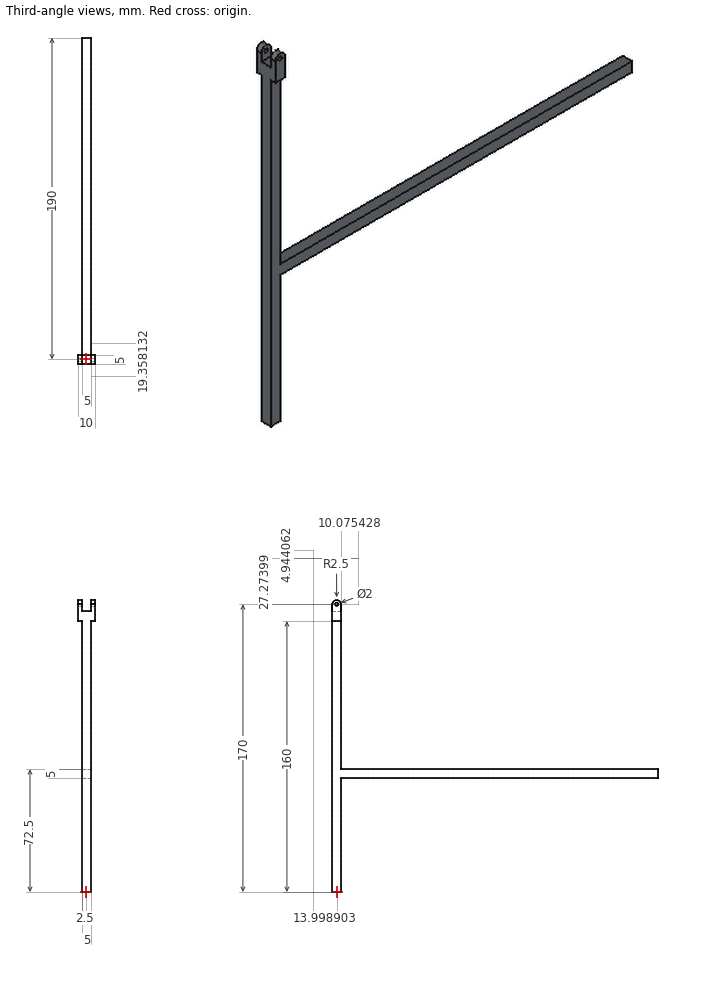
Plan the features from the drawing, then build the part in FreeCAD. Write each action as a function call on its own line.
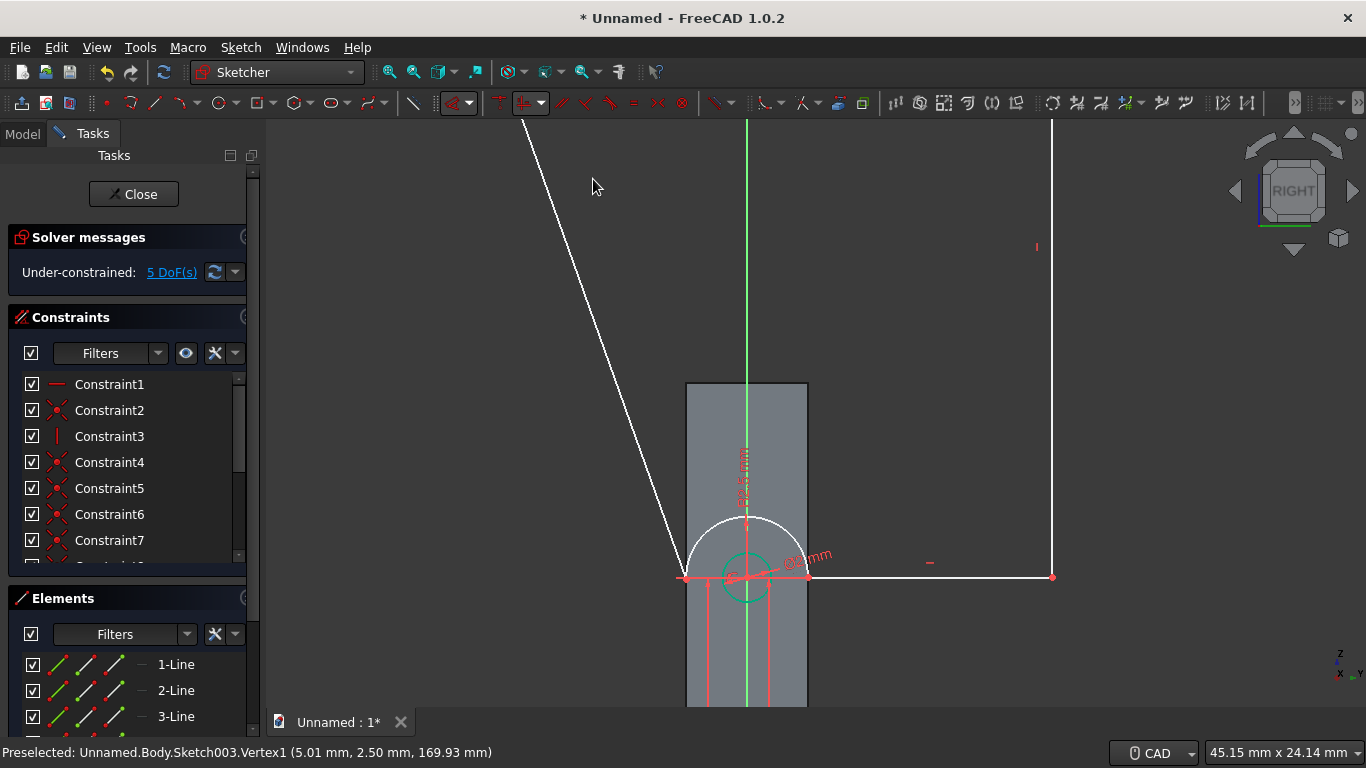
click(686, 579)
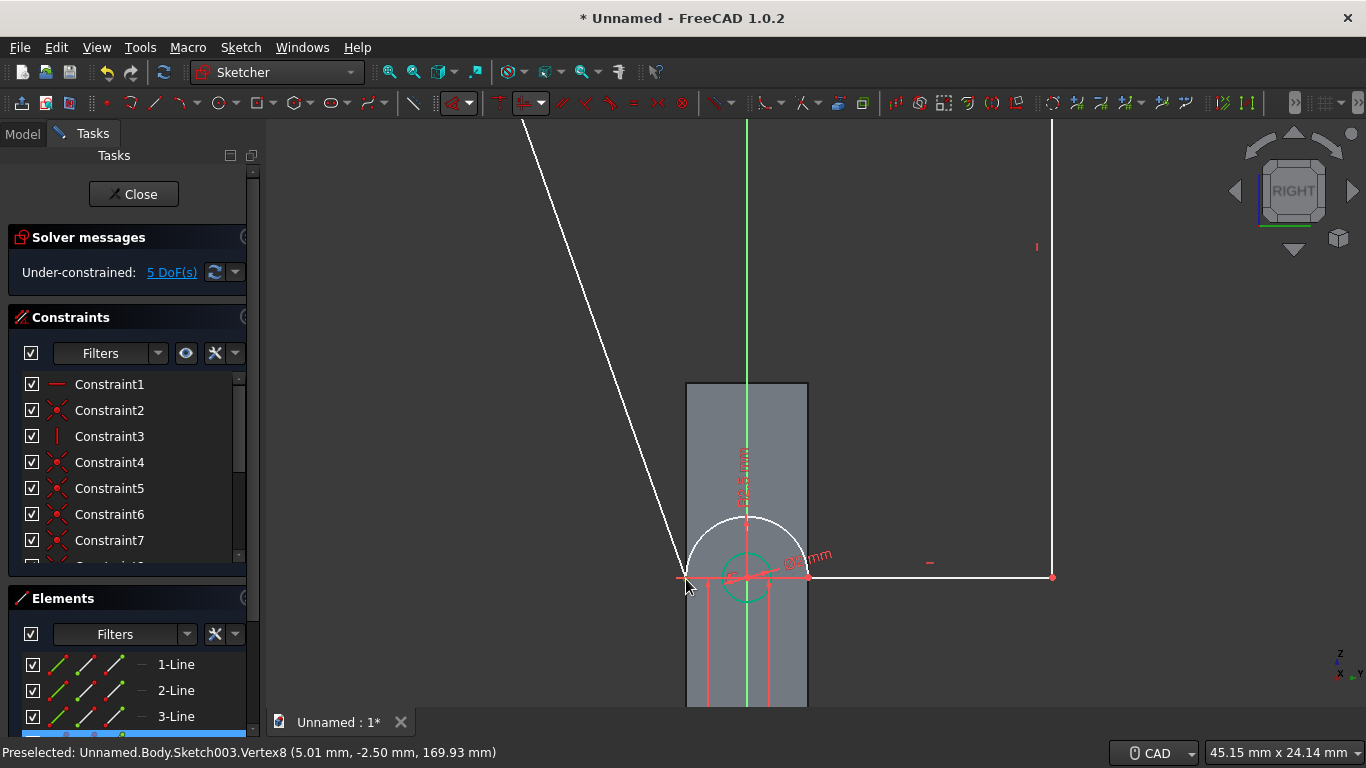
click(472, 104)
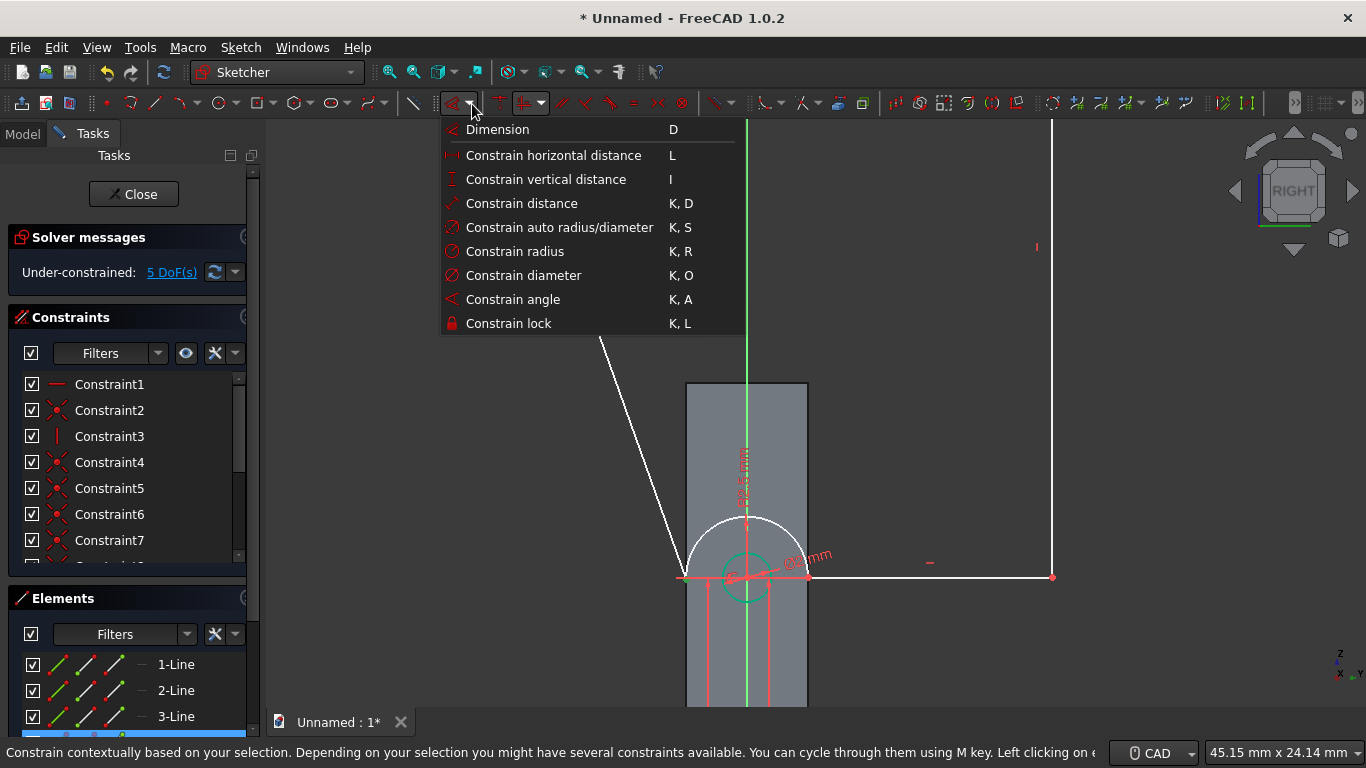
click(593, 179)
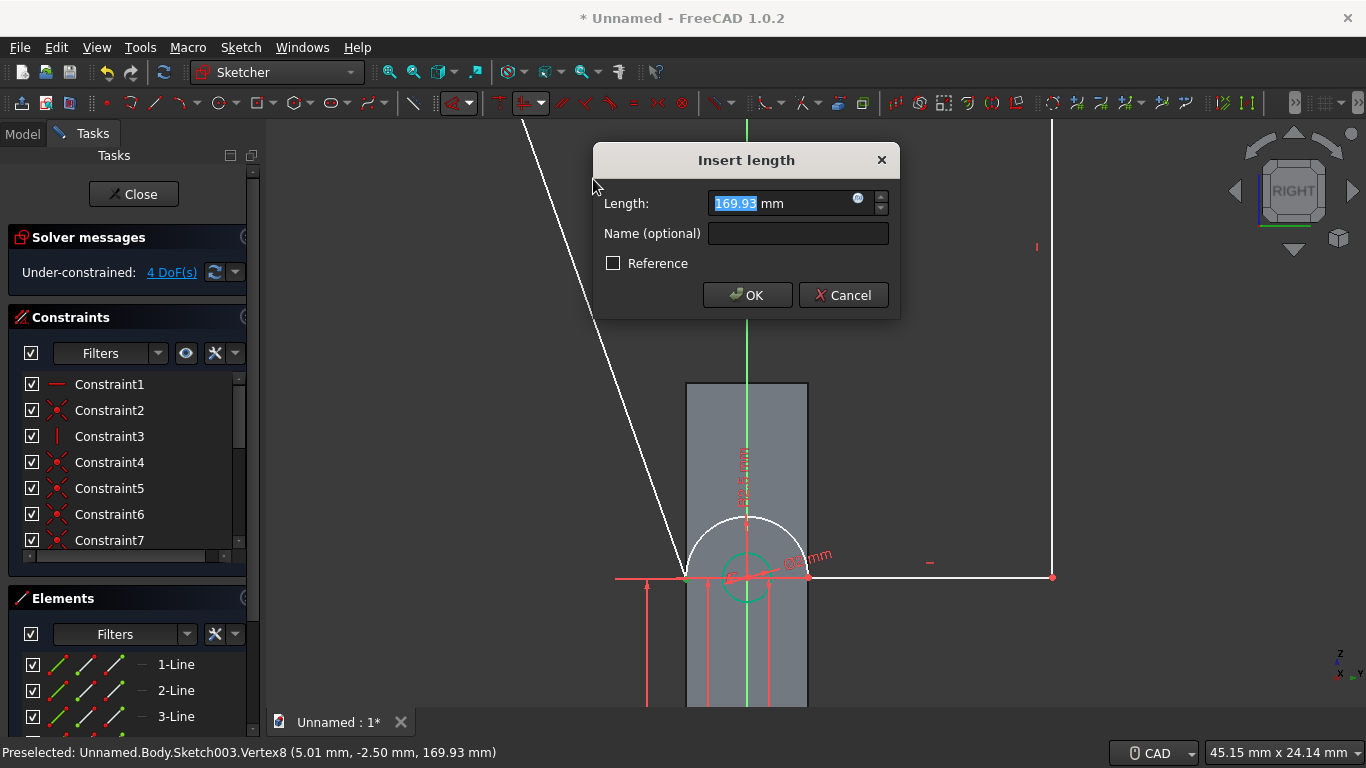
text(170)
key(Return)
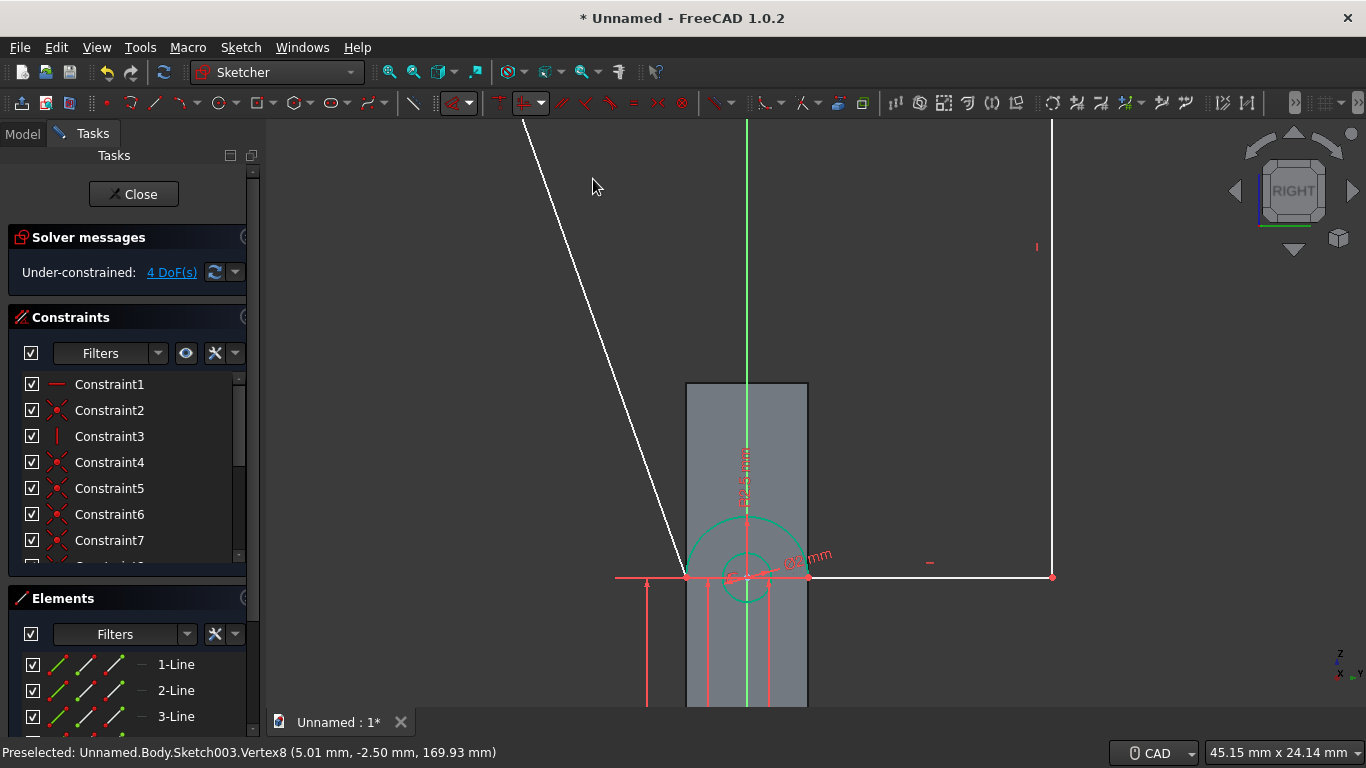
click(1052, 379)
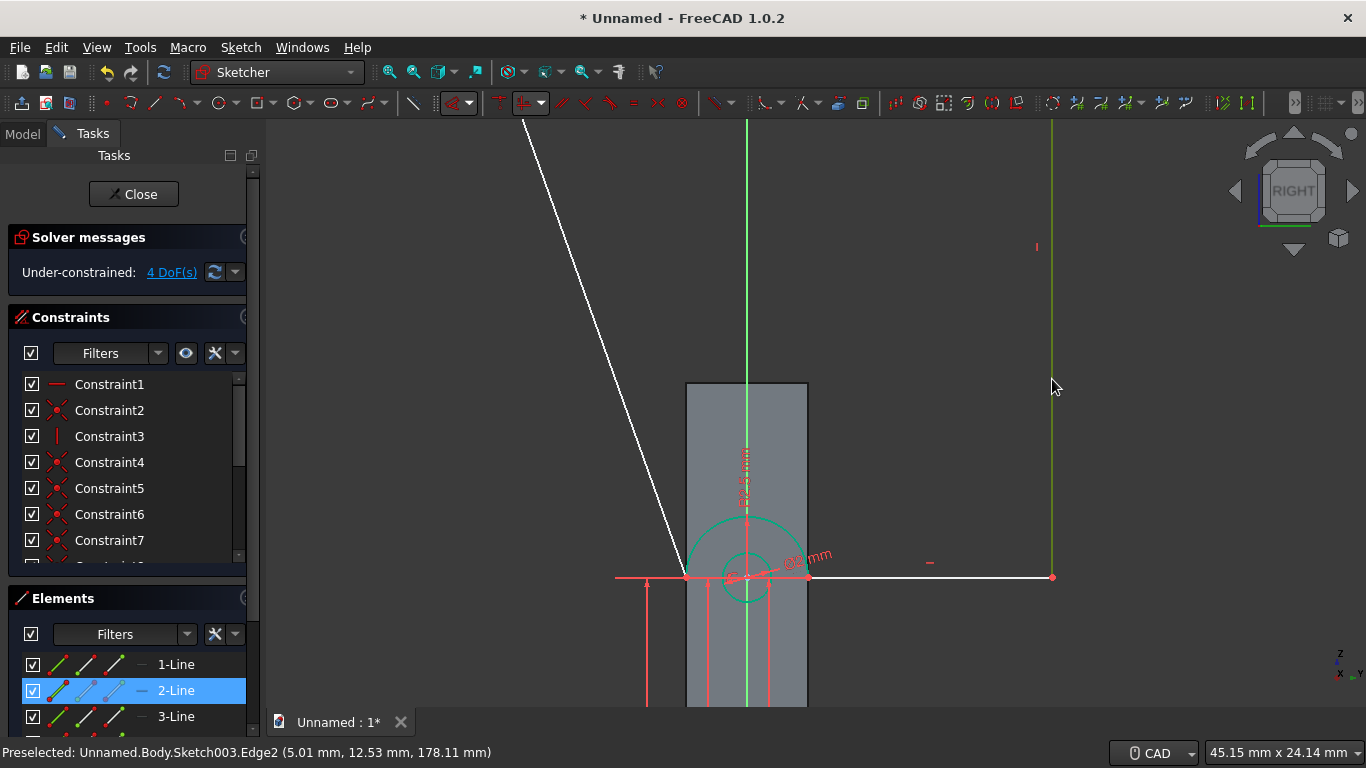
click(472, 104)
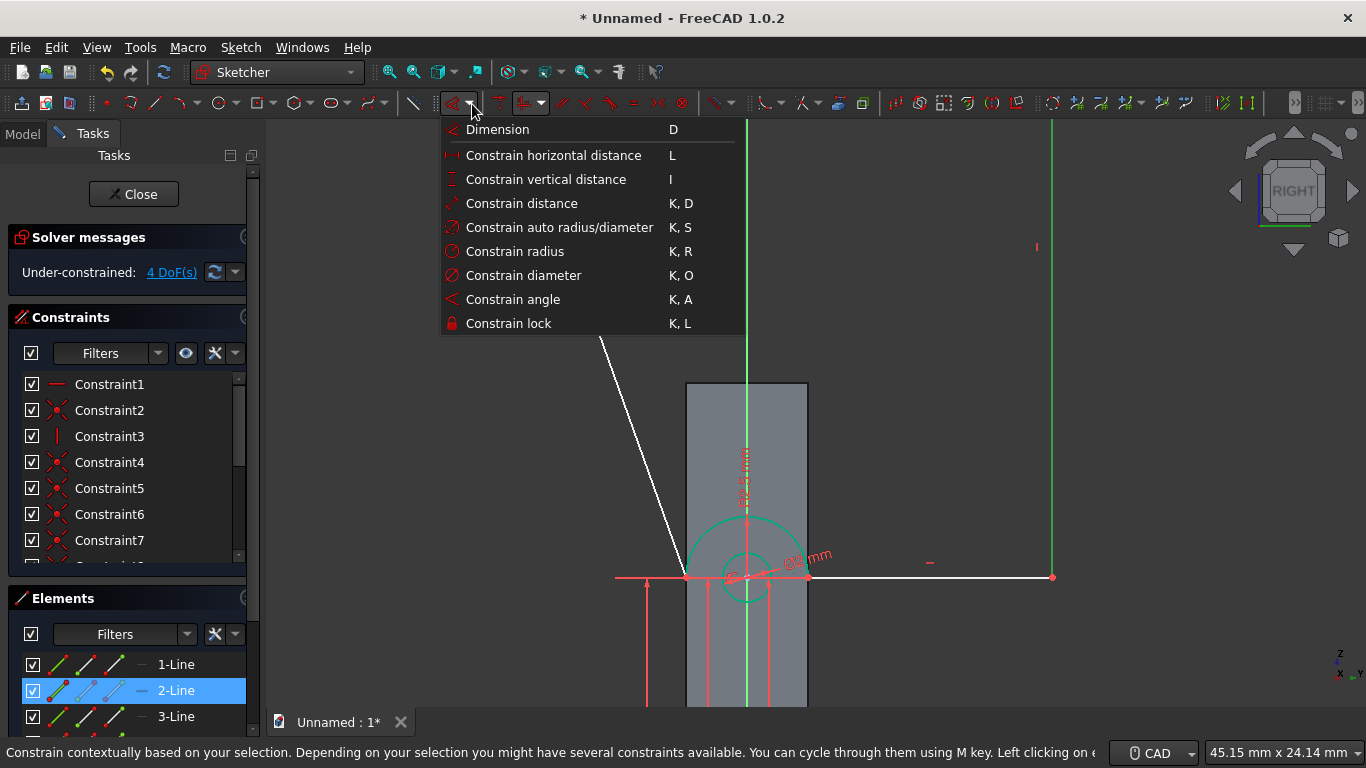
click(593, 179)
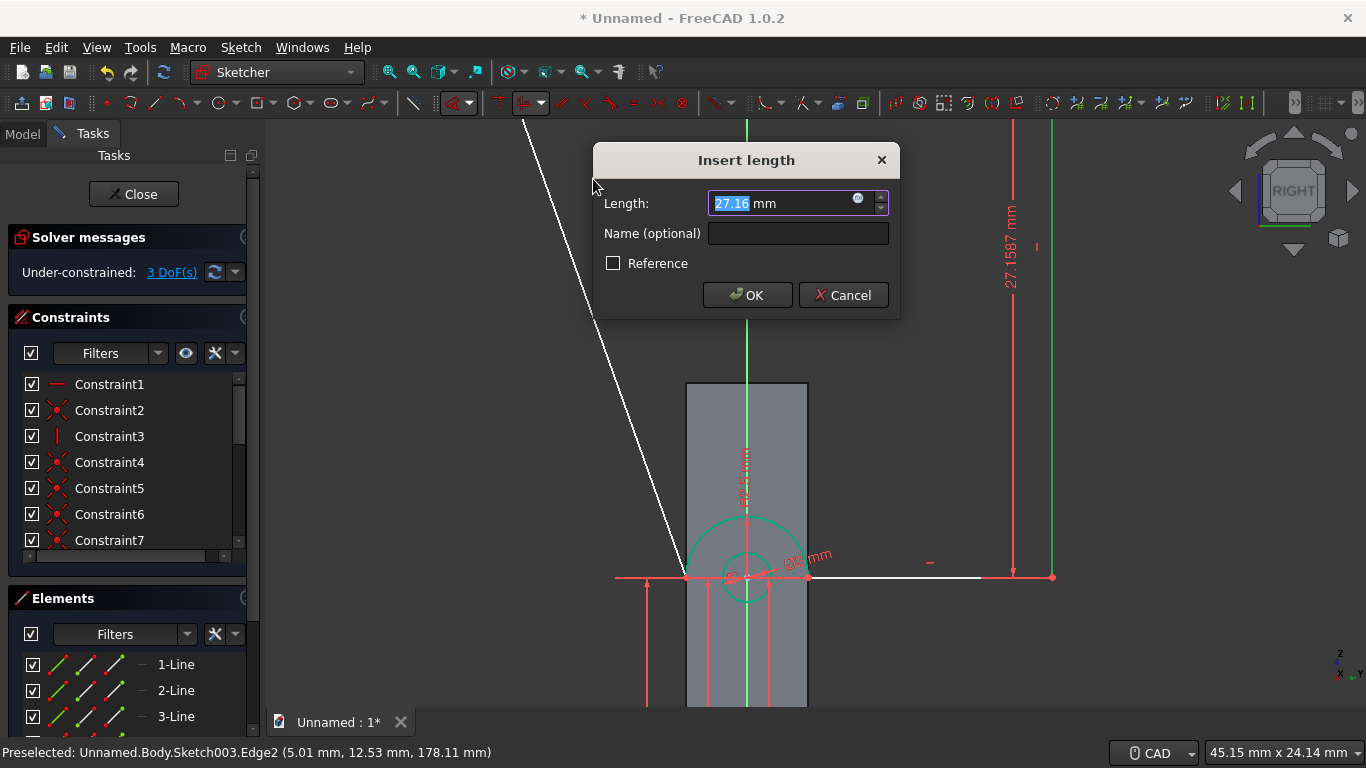
text(27.27399)
key(Return)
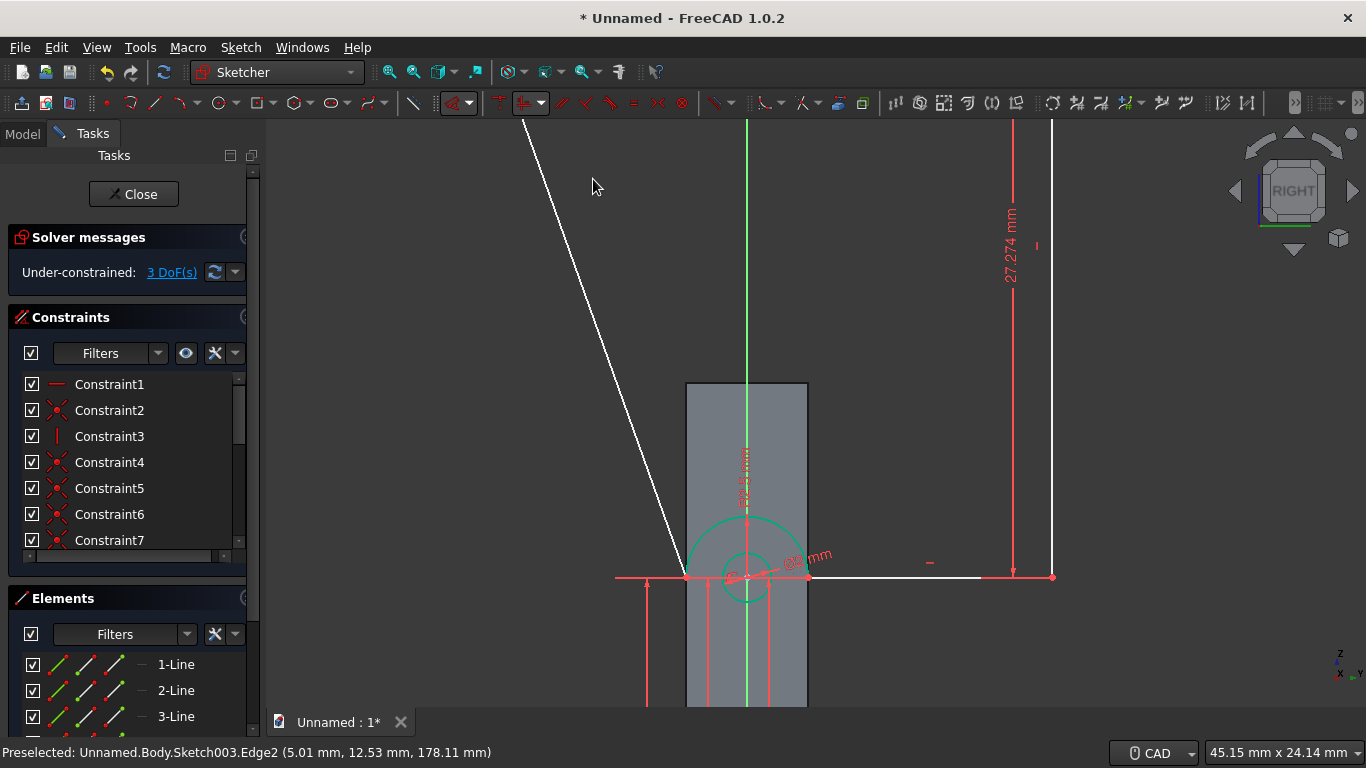
click(881, 578)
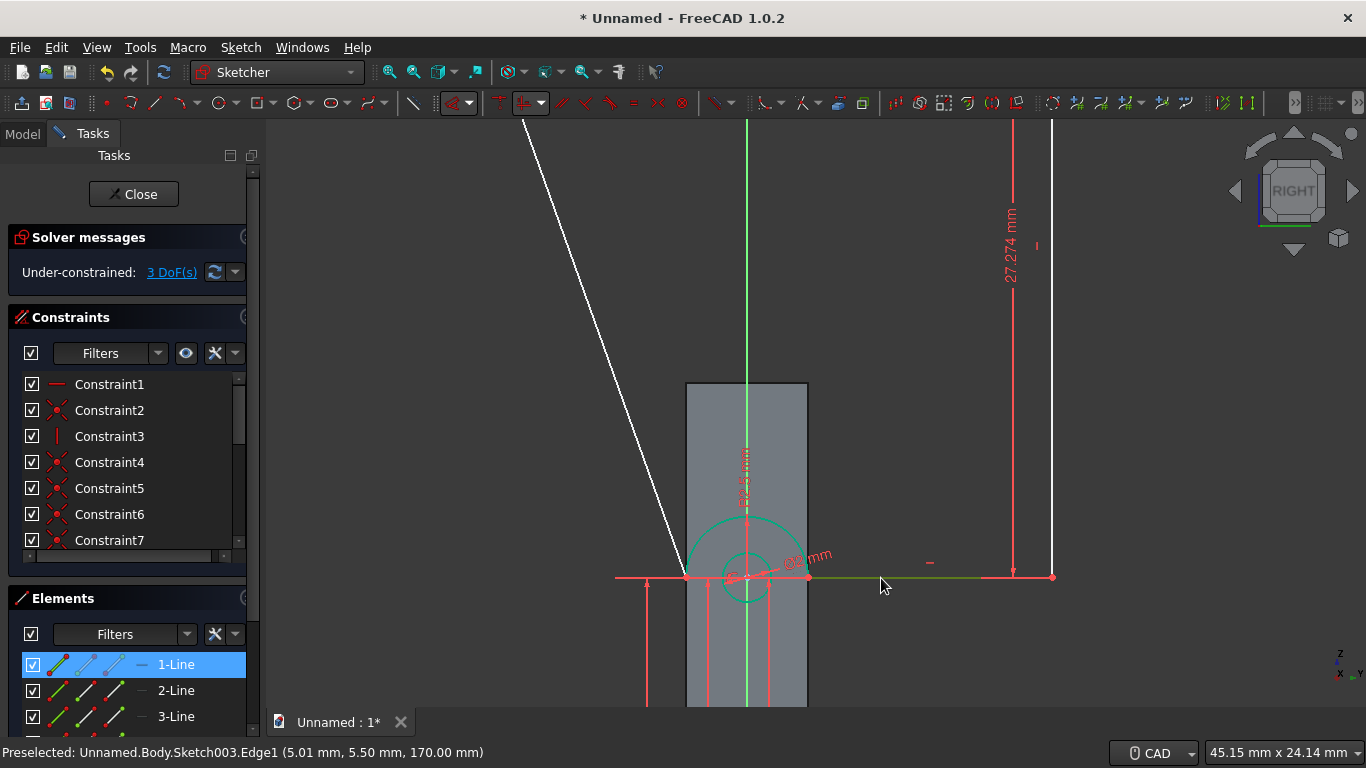
key(l)